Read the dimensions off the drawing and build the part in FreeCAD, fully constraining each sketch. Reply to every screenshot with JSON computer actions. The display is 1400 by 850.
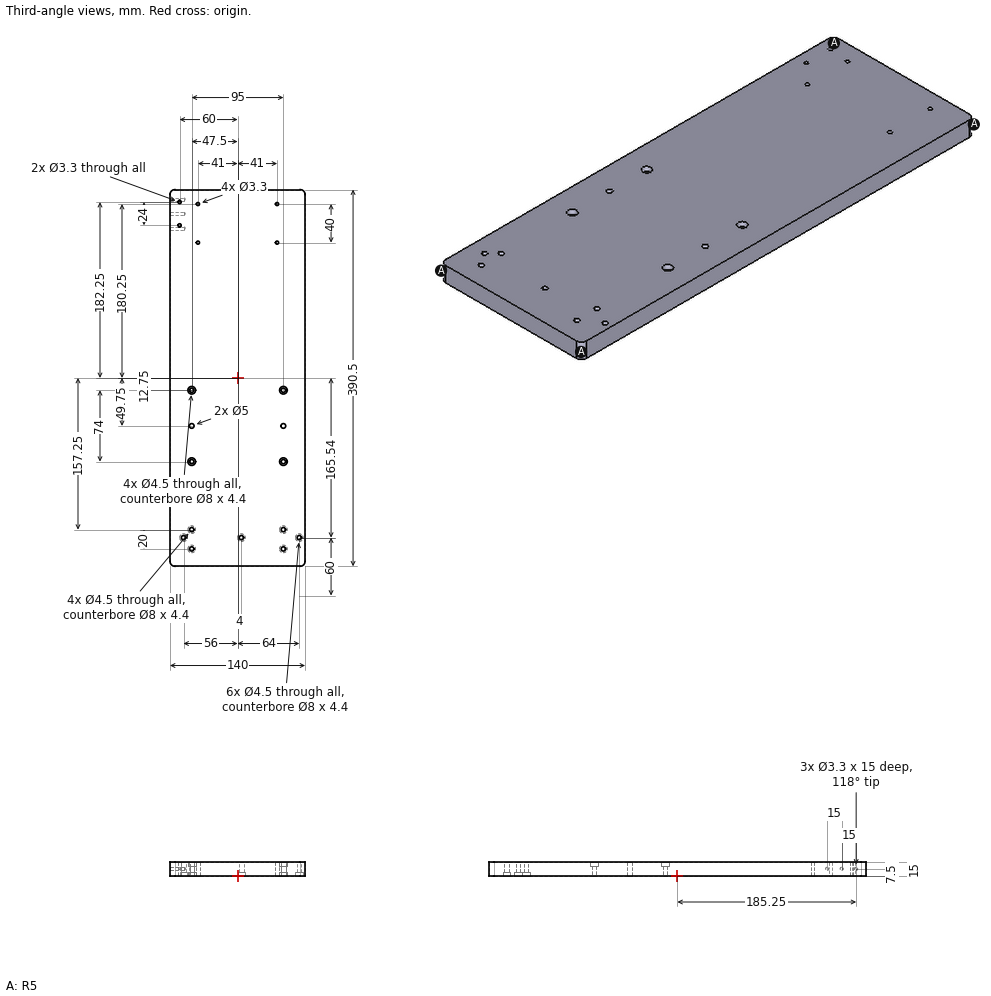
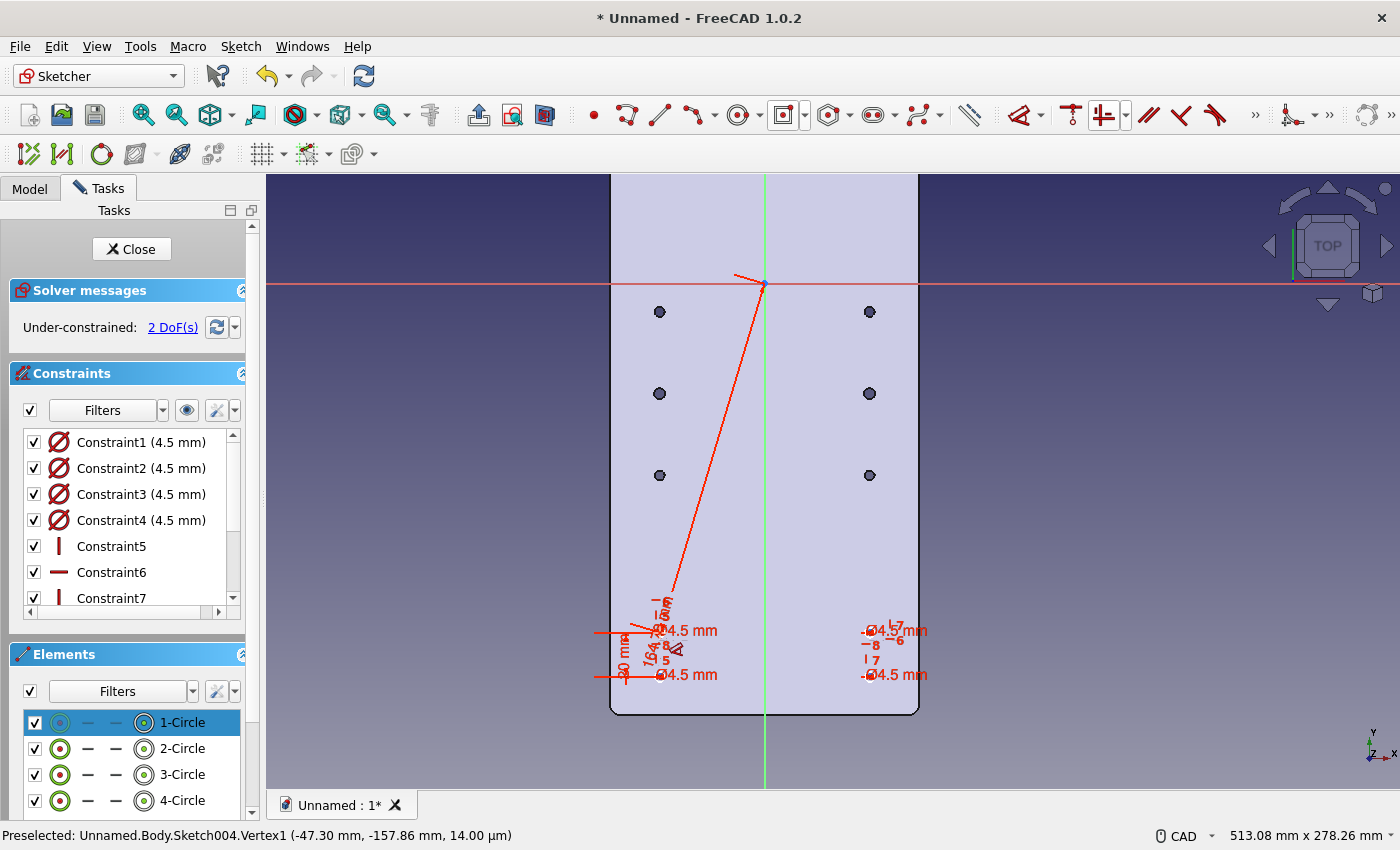
{"action": "left_click", "coordinate": [870, 633]}
{"action": "left_click", "coordinate": [717, 667]}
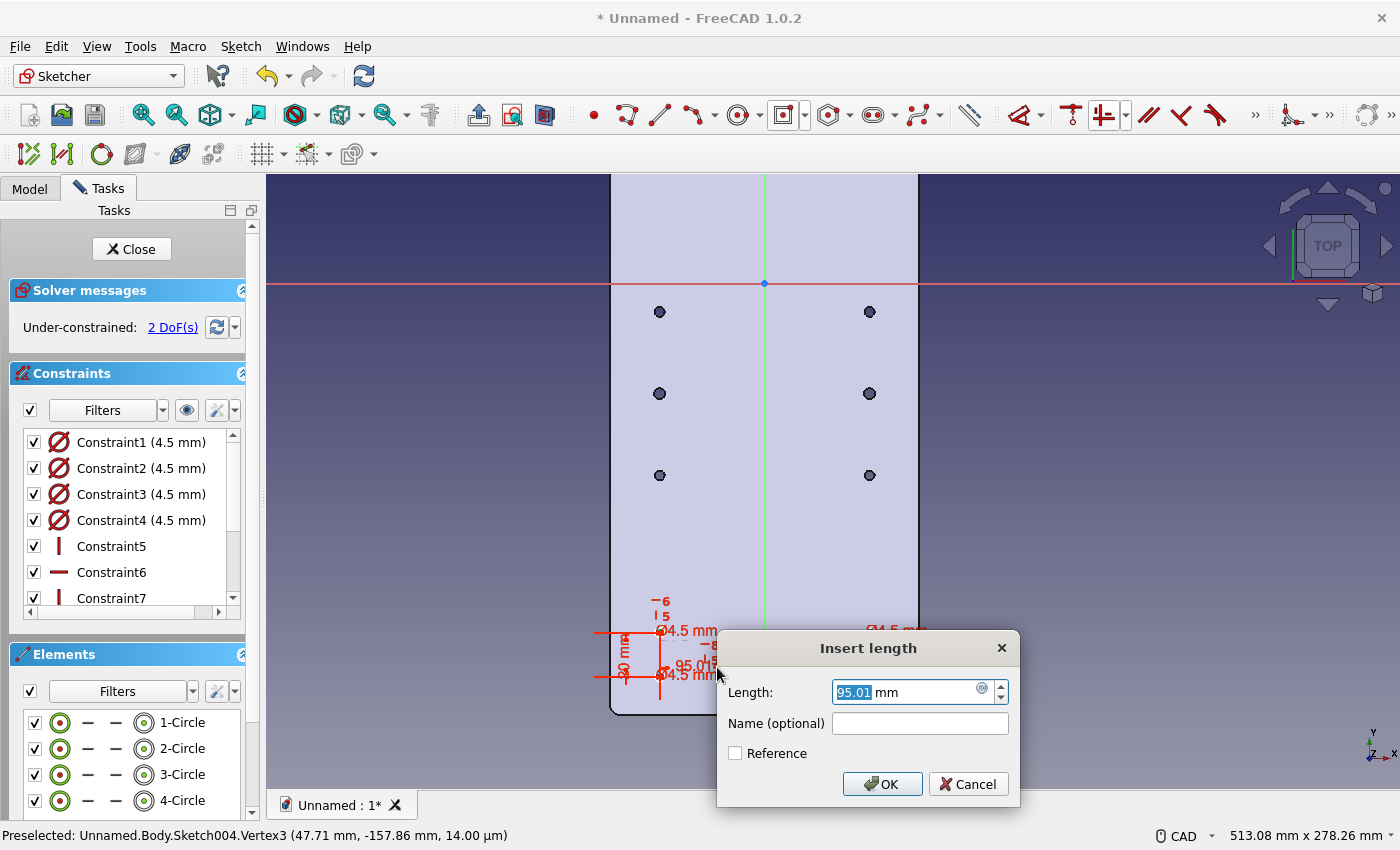
{"action": "type", "text": "95"}
{"action": "key", "text": "Return"}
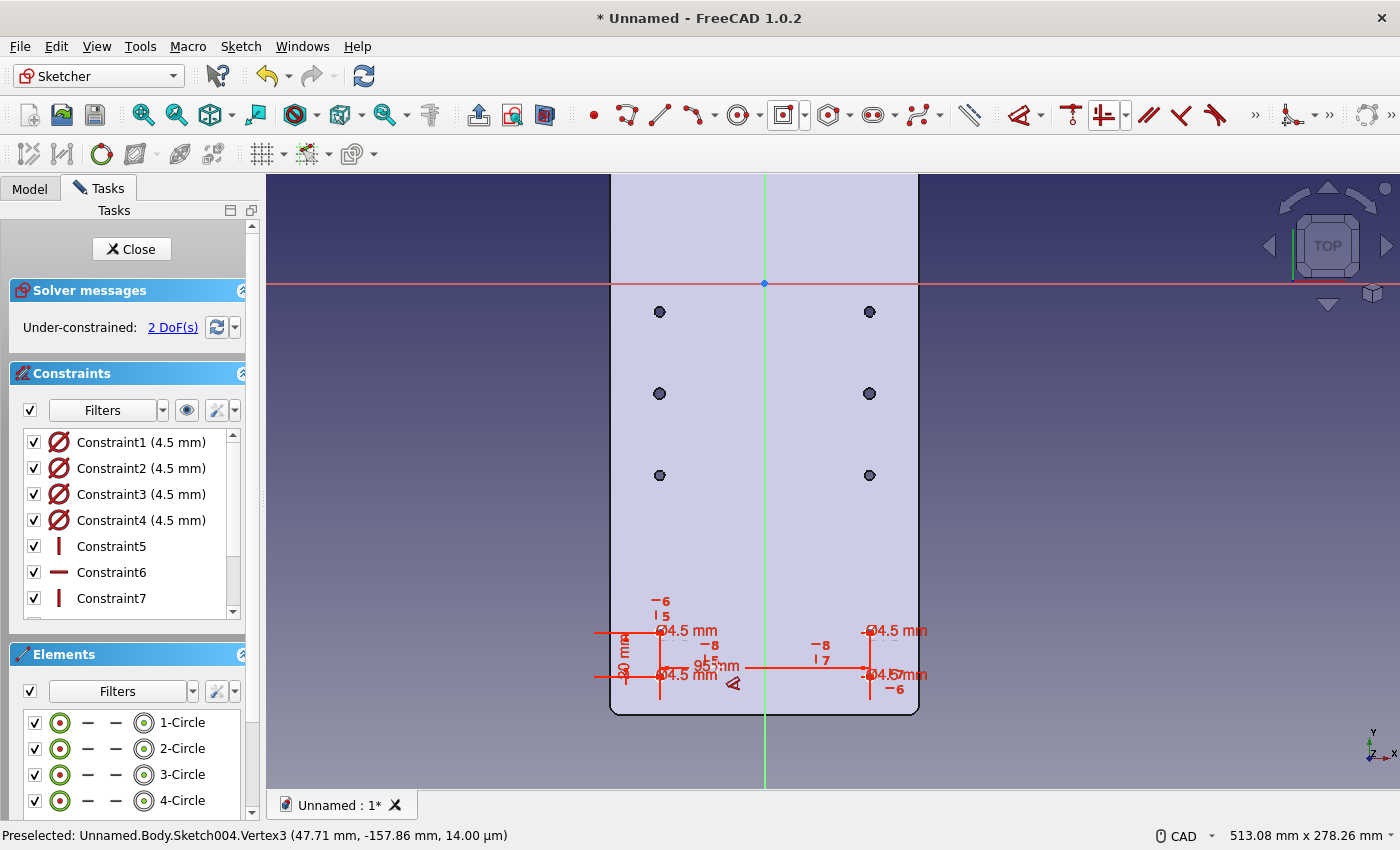
{"action": "left_click", "coordinate": [660, 633]}
{"action": "left_click", "coordinate": [712, 250]}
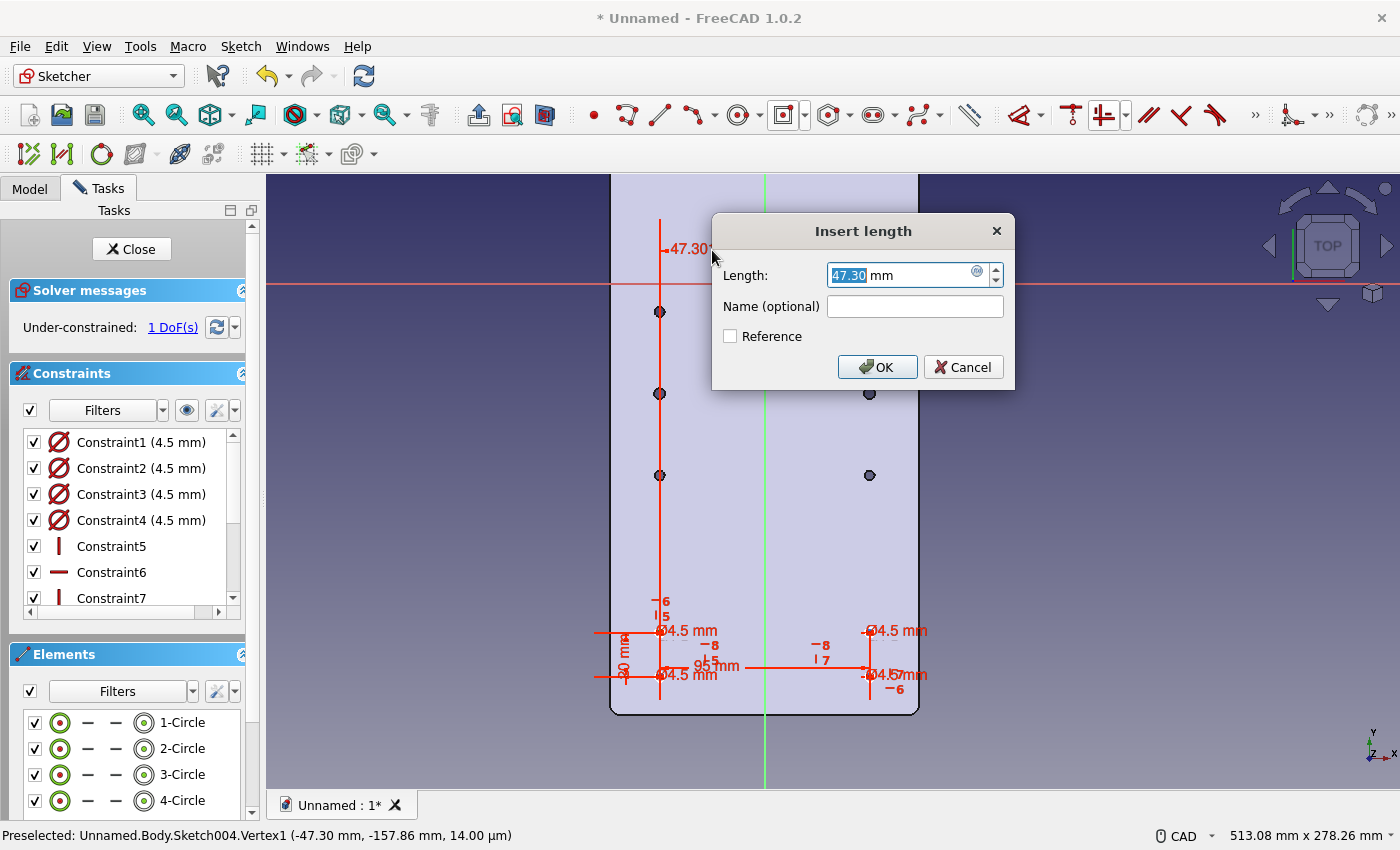
{"action": "type", "text": "47.5"}
{"action": "key", "text": "Return"}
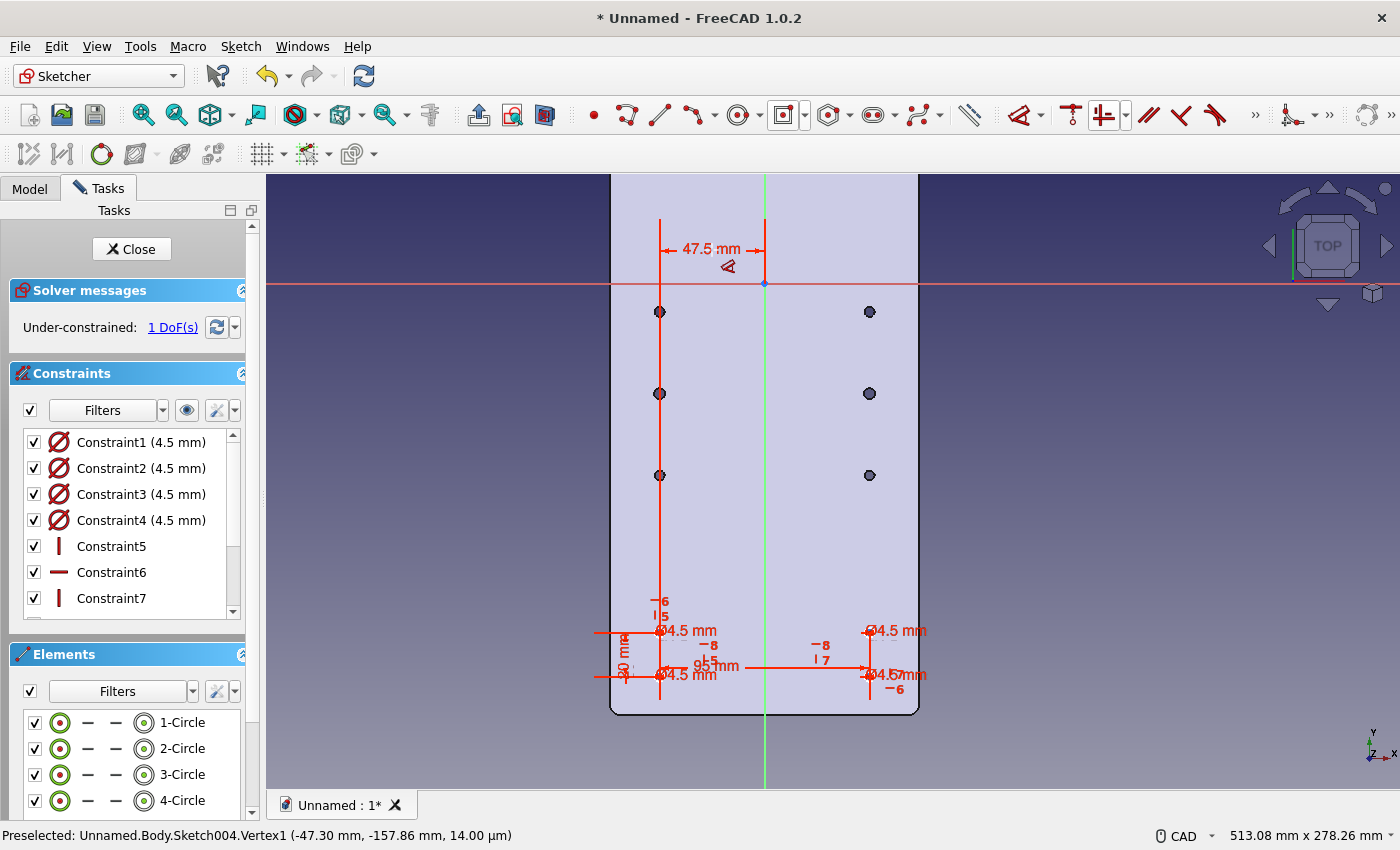
{"action": "left_click", "coordinate": [660, 633]}
{"action": "left_click", "coordinate": [626, 458]}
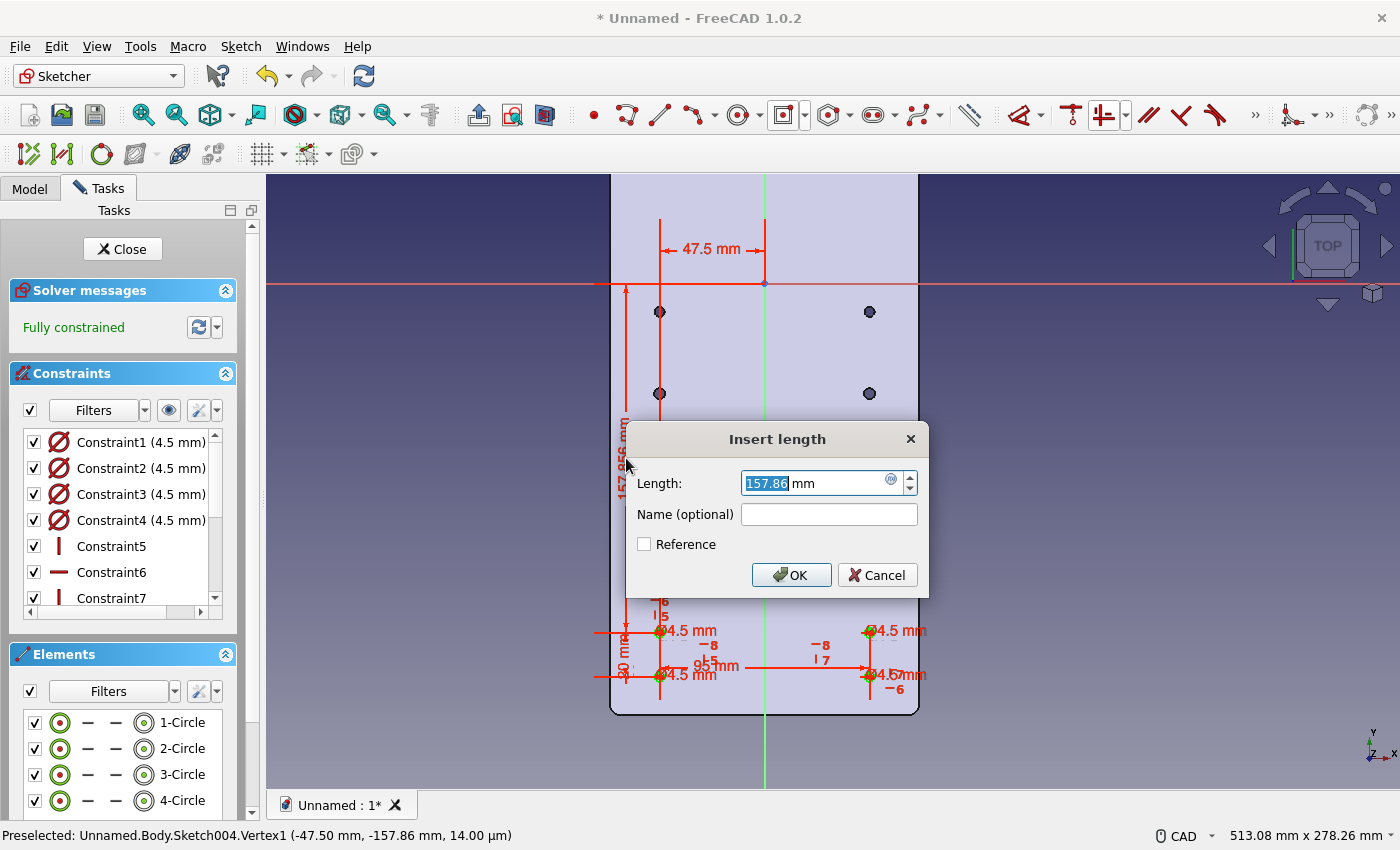
{"action": "type", "text": "157.25"}
{"action": "key", "text": "Return"}
{"action": "key", "text": "Escape"}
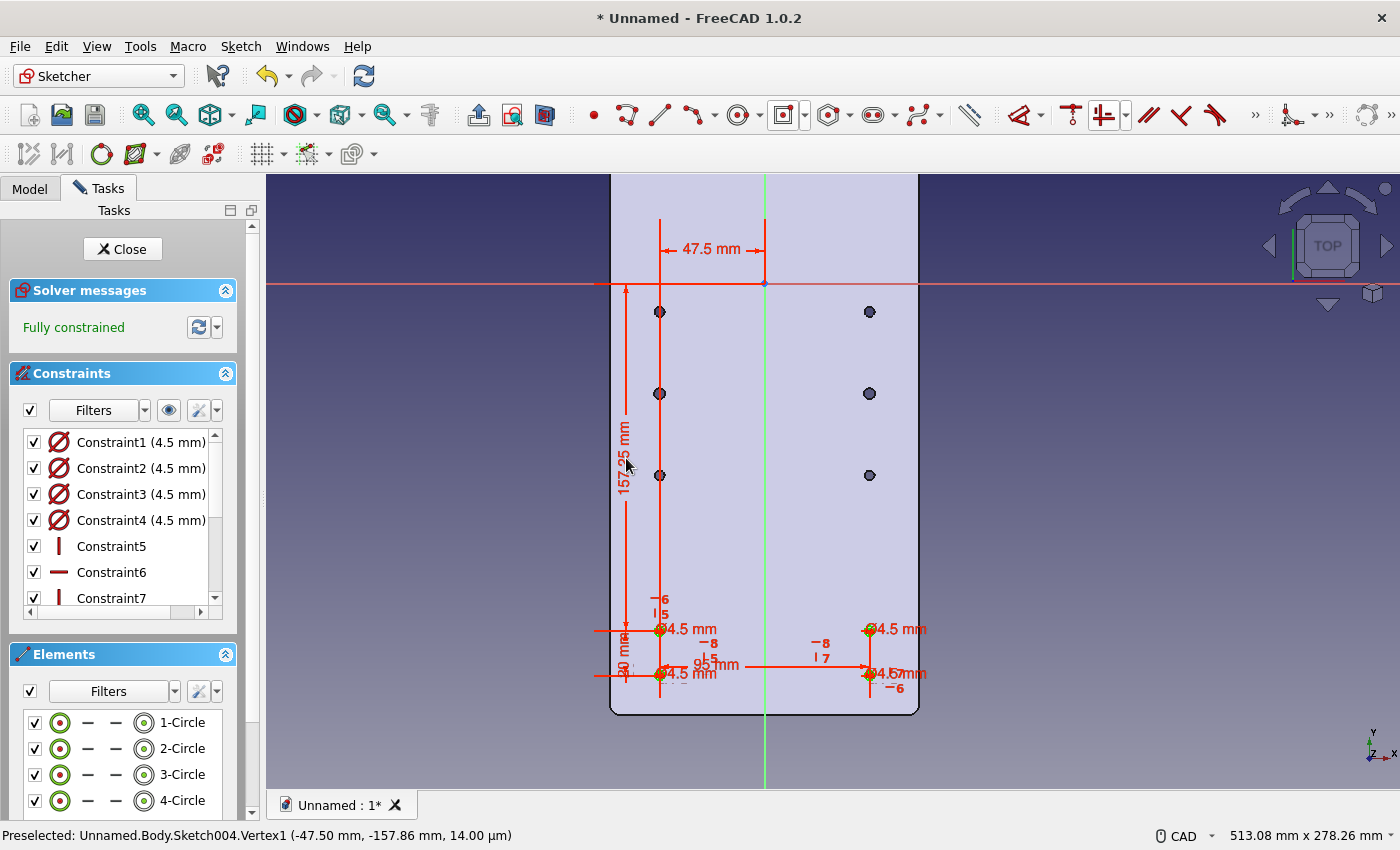
{"action": "left_click", "coordinate": [123, 249]}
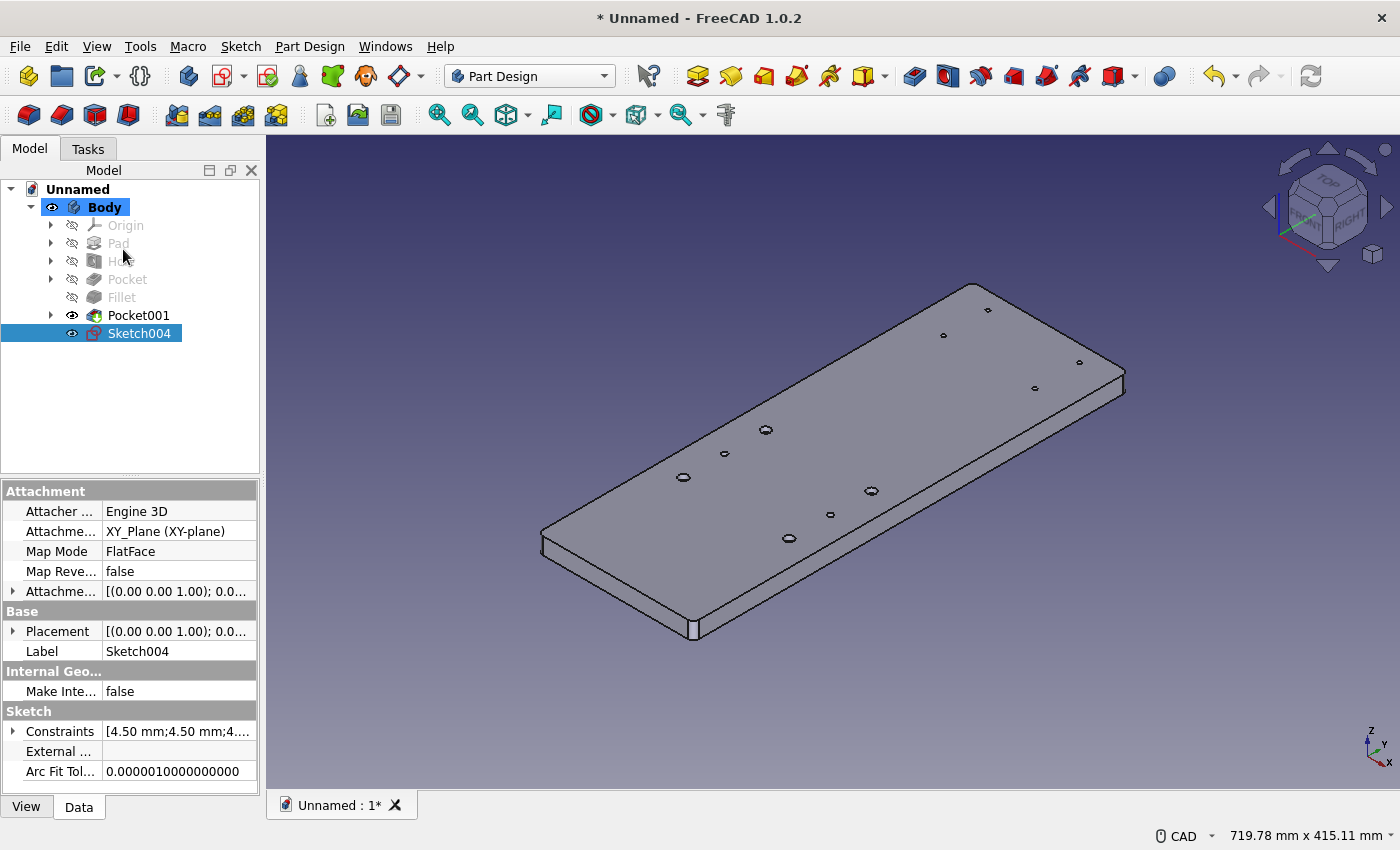
{"action": "left_click", "coordinate": [948, 76]}